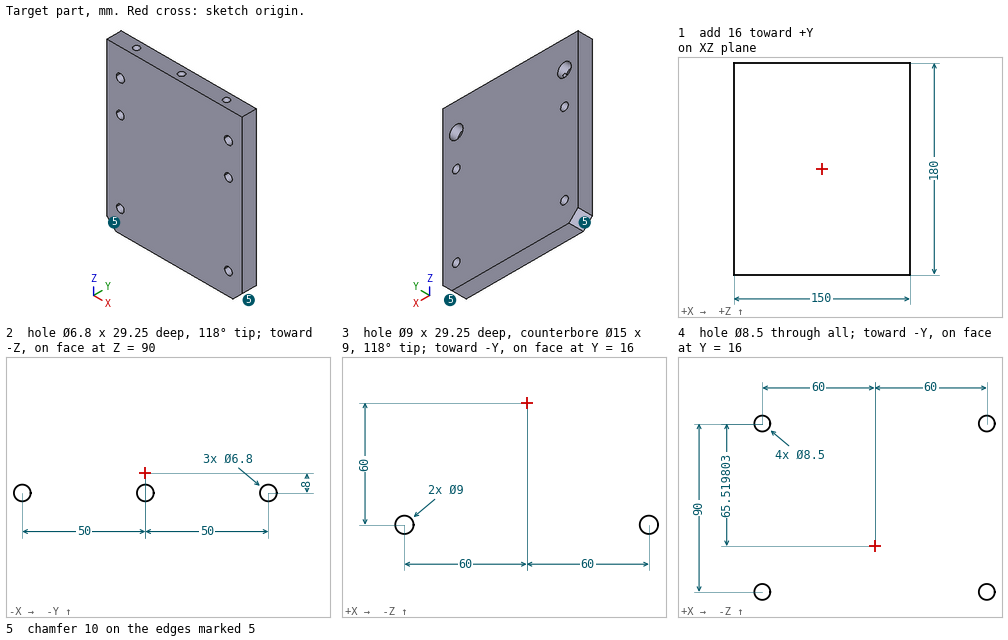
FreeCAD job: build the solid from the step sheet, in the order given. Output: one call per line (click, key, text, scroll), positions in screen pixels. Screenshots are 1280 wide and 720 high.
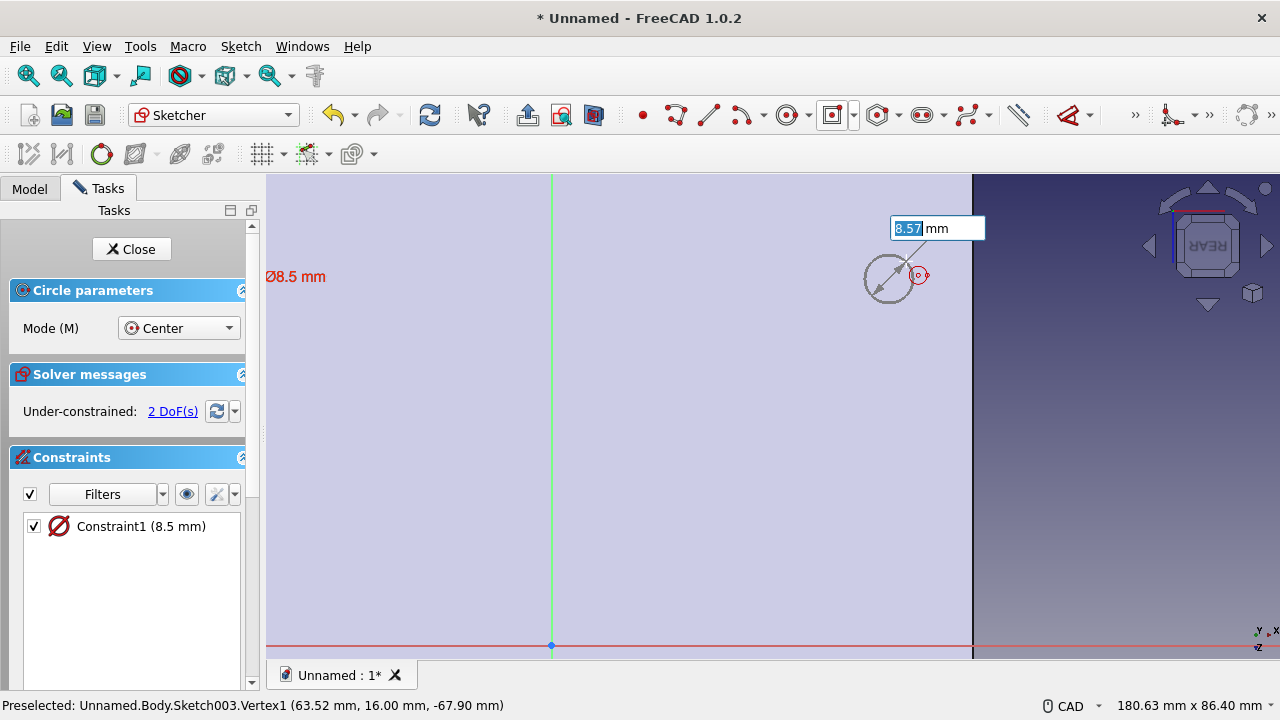
text(8.5)
key(Return)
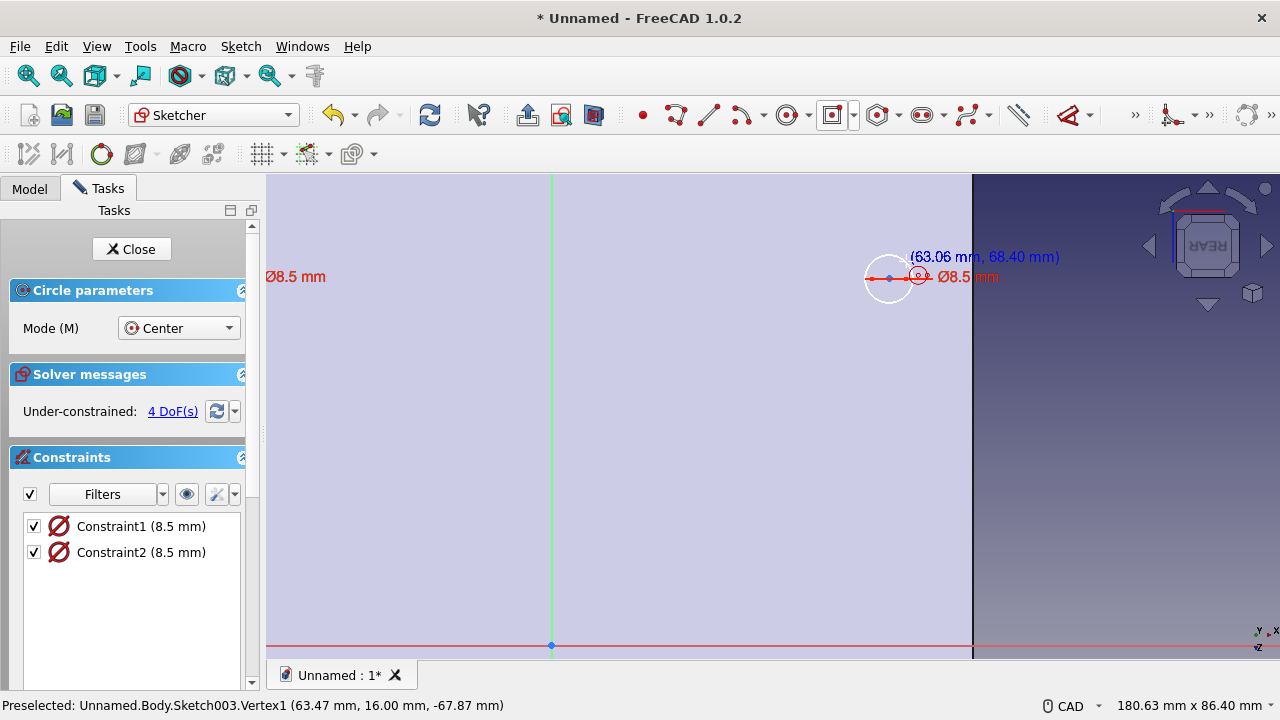
scroll(890, 278, down, 3)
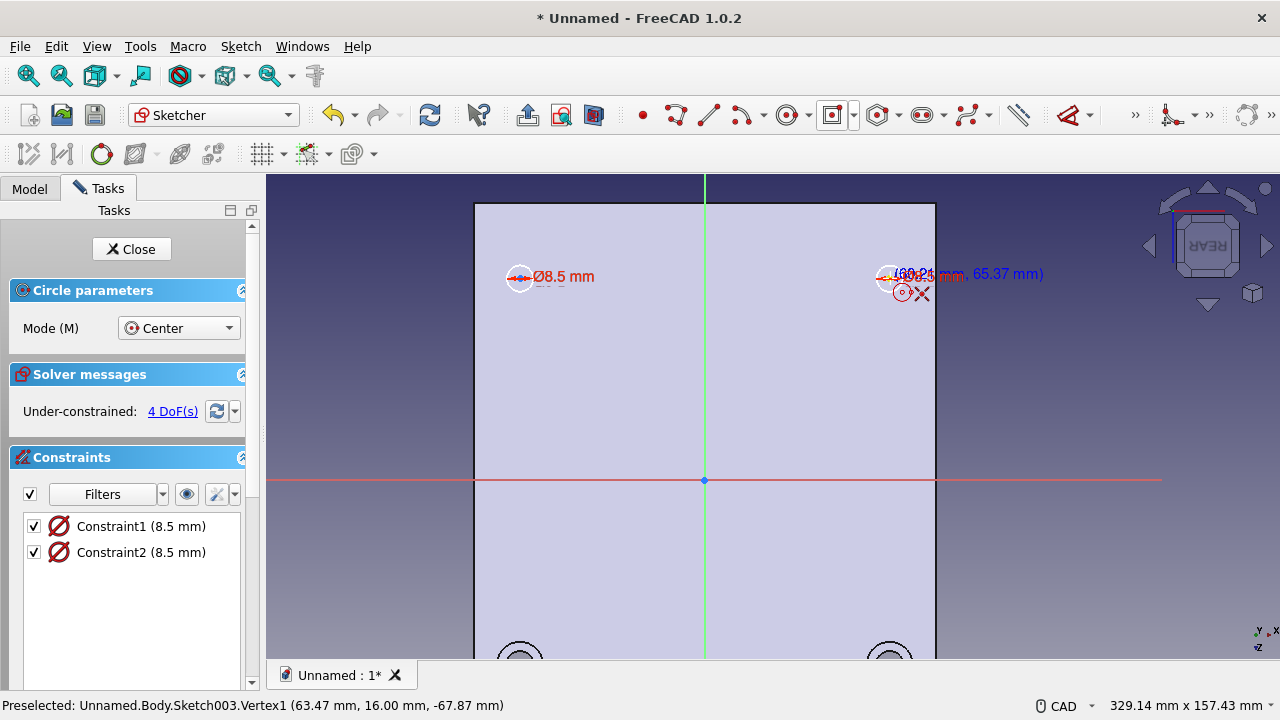
scroll(520, 555, up, 3)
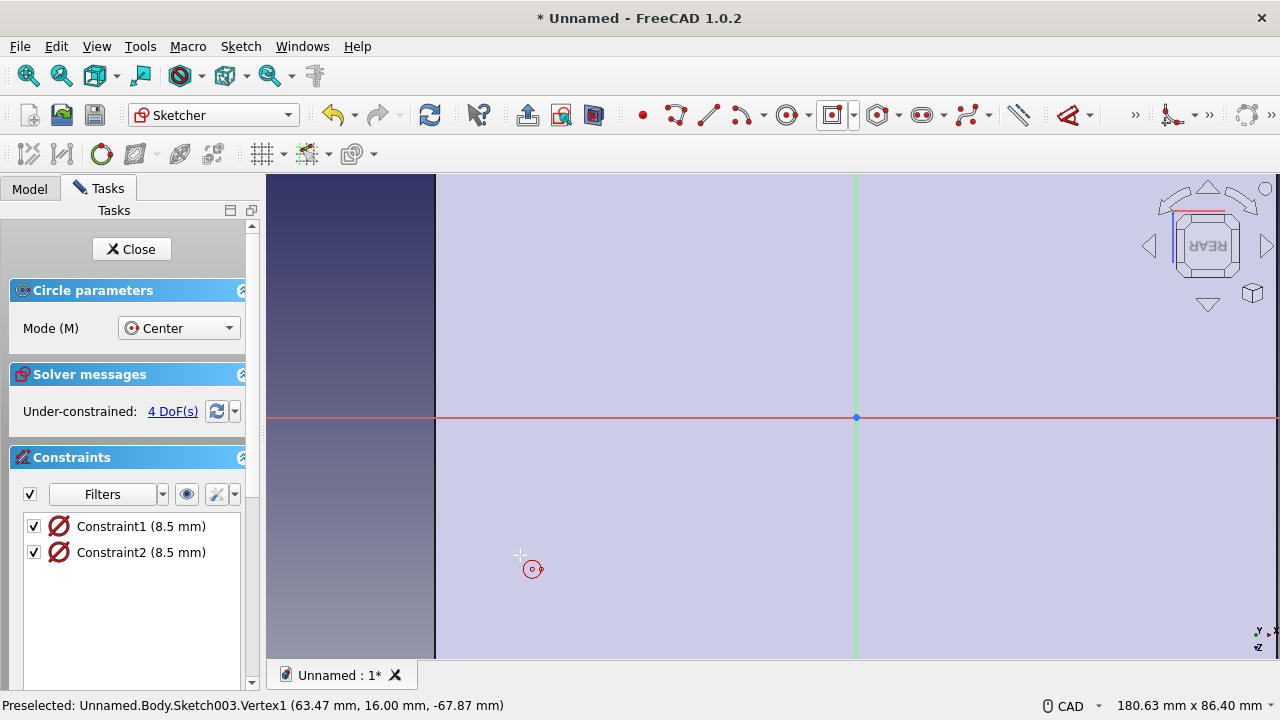
click(520, 555)
move(537, 538)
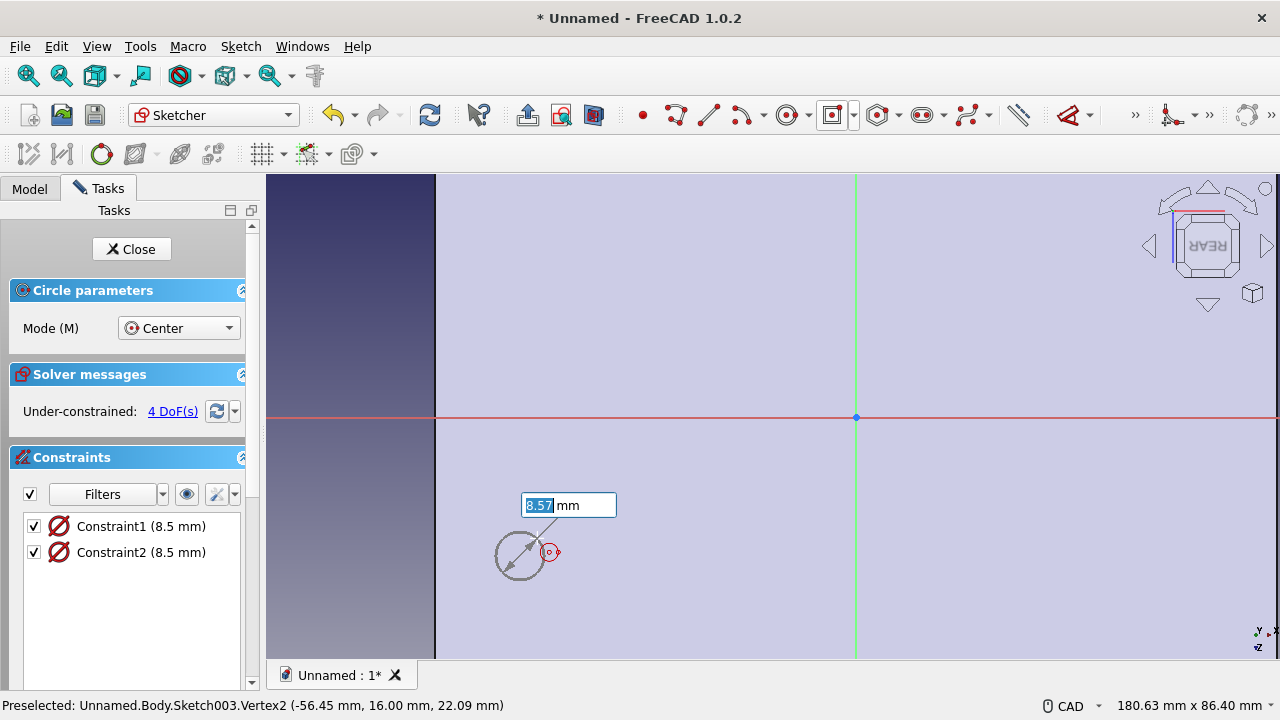
text(8.5)
key(Return)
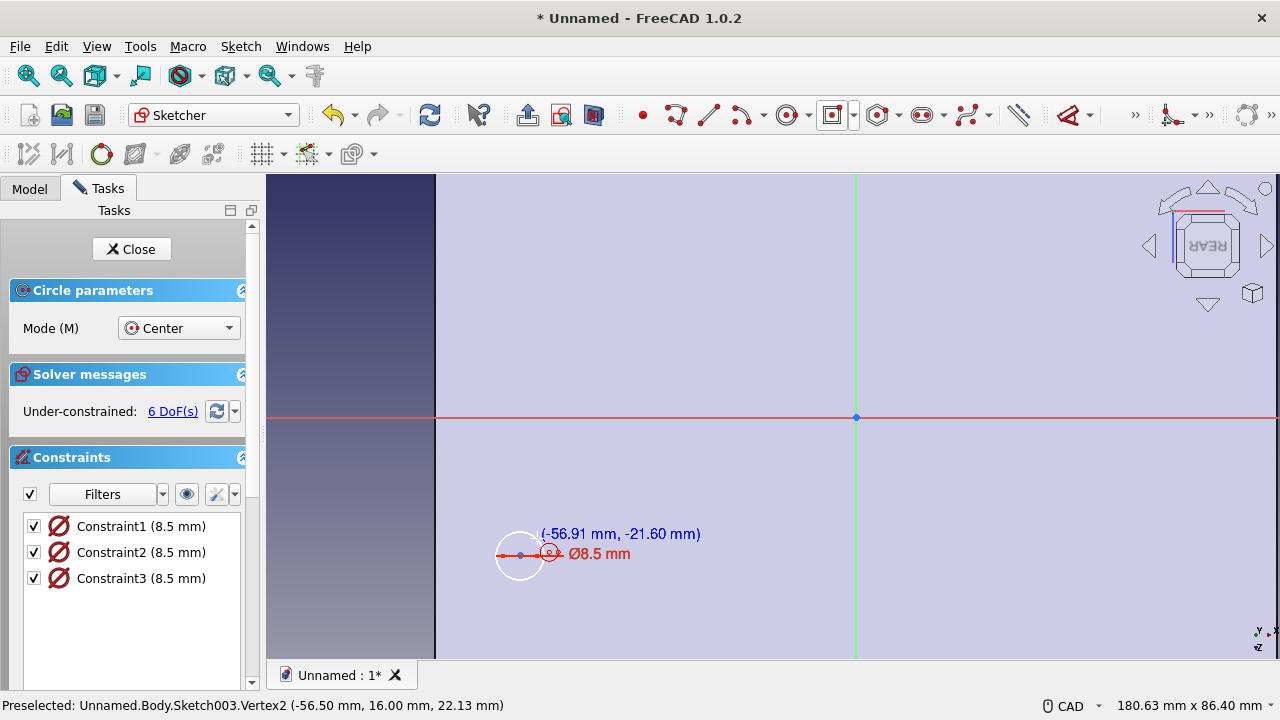
scroll(520, 555, down, 3)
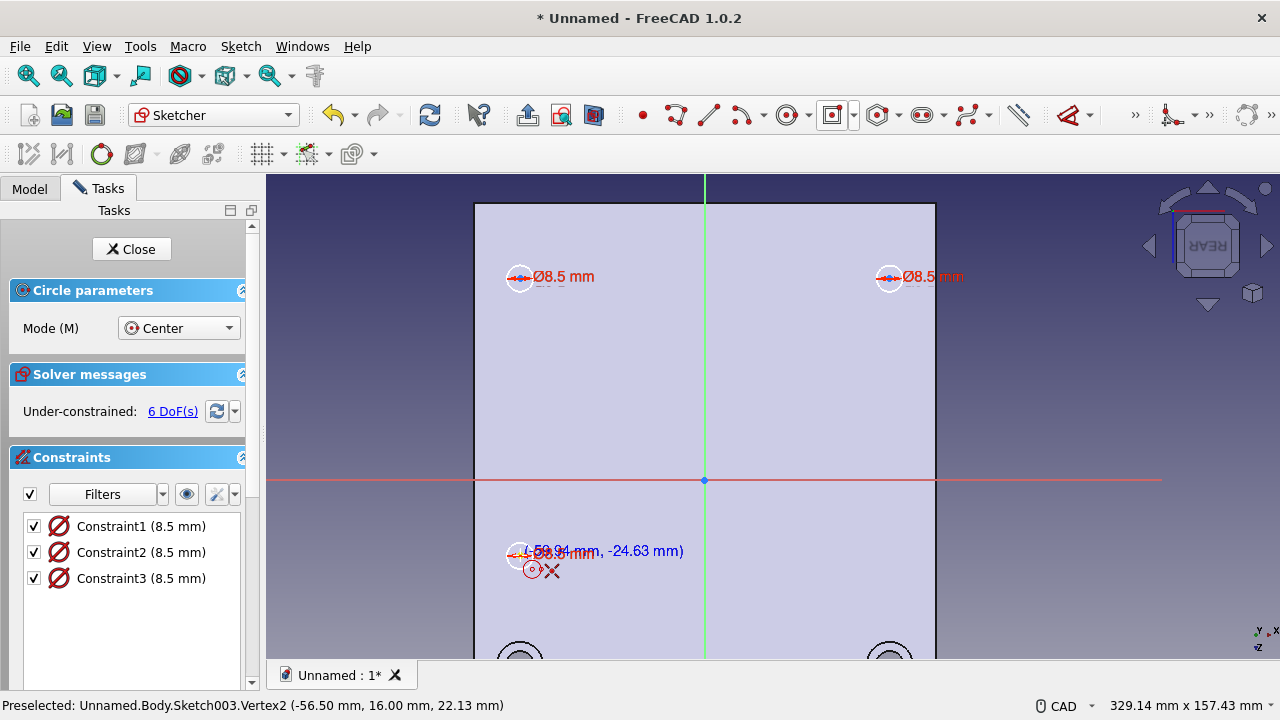
scroll(890, 555, up, 3)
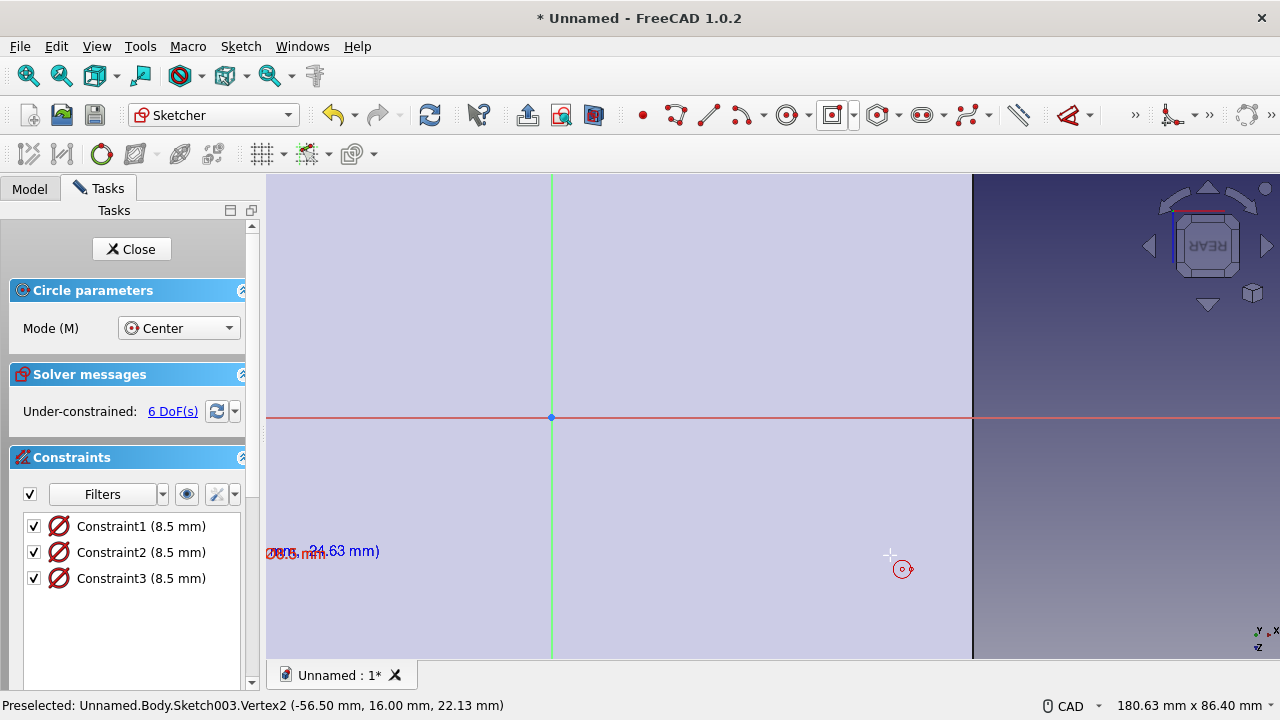
click(889, 555)
move(906, 538)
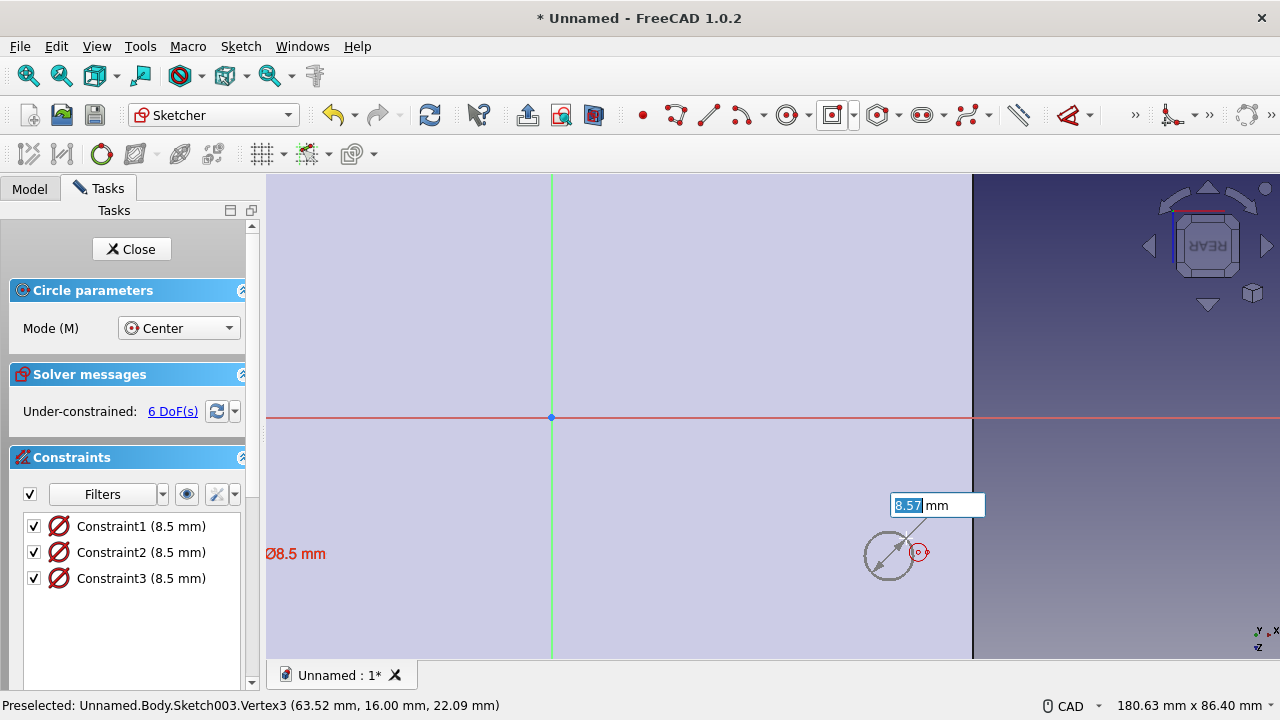
text(8.5)
key(Return)
key(Escape)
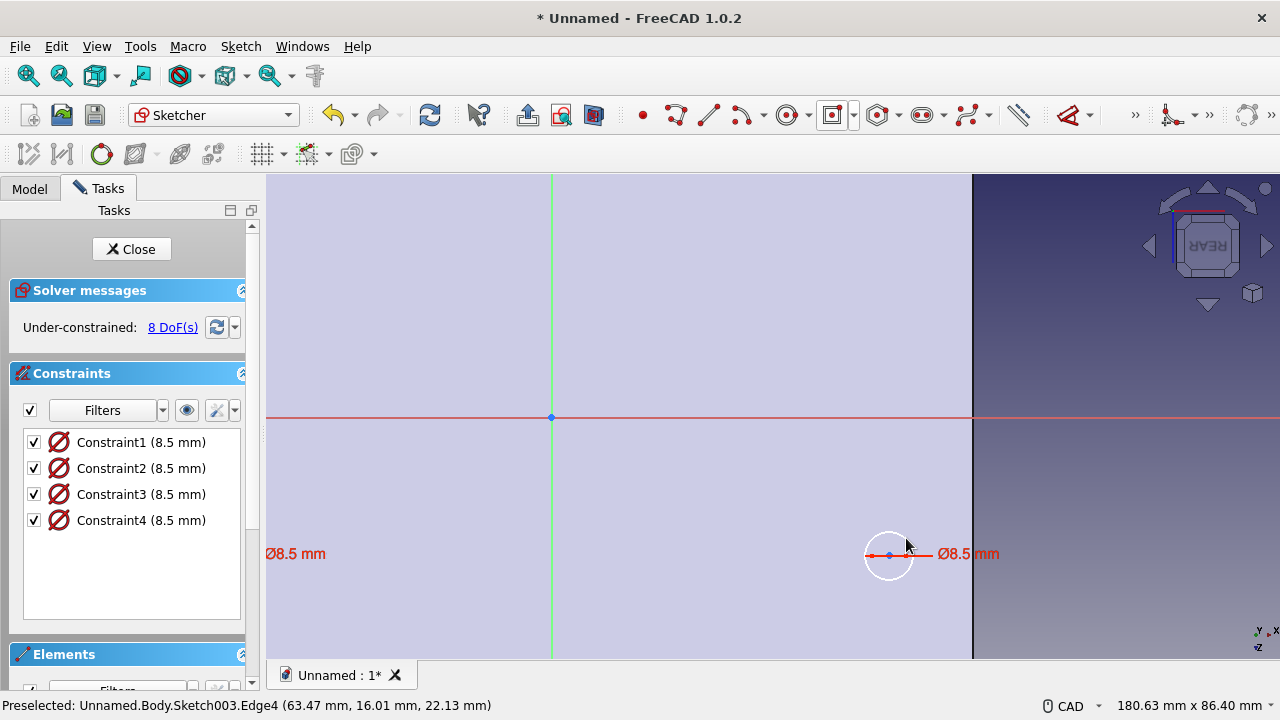
scroll(890, 555, down, 3)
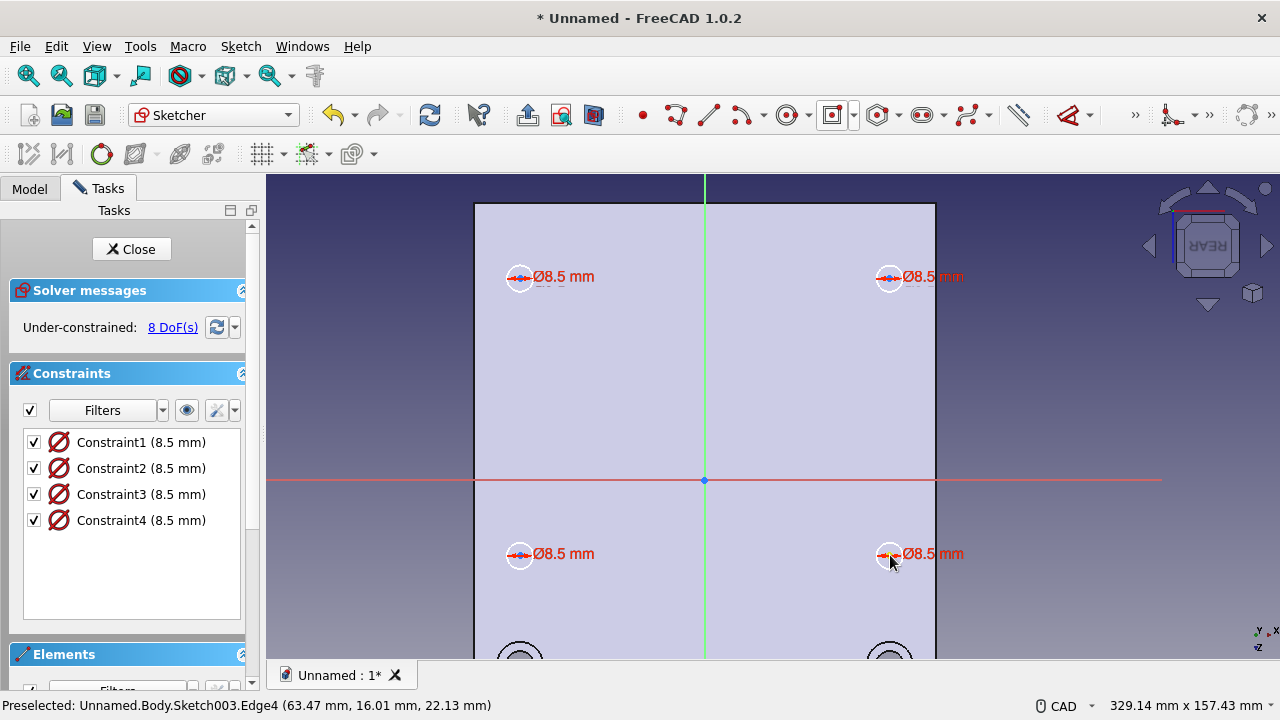
click(520, 279)